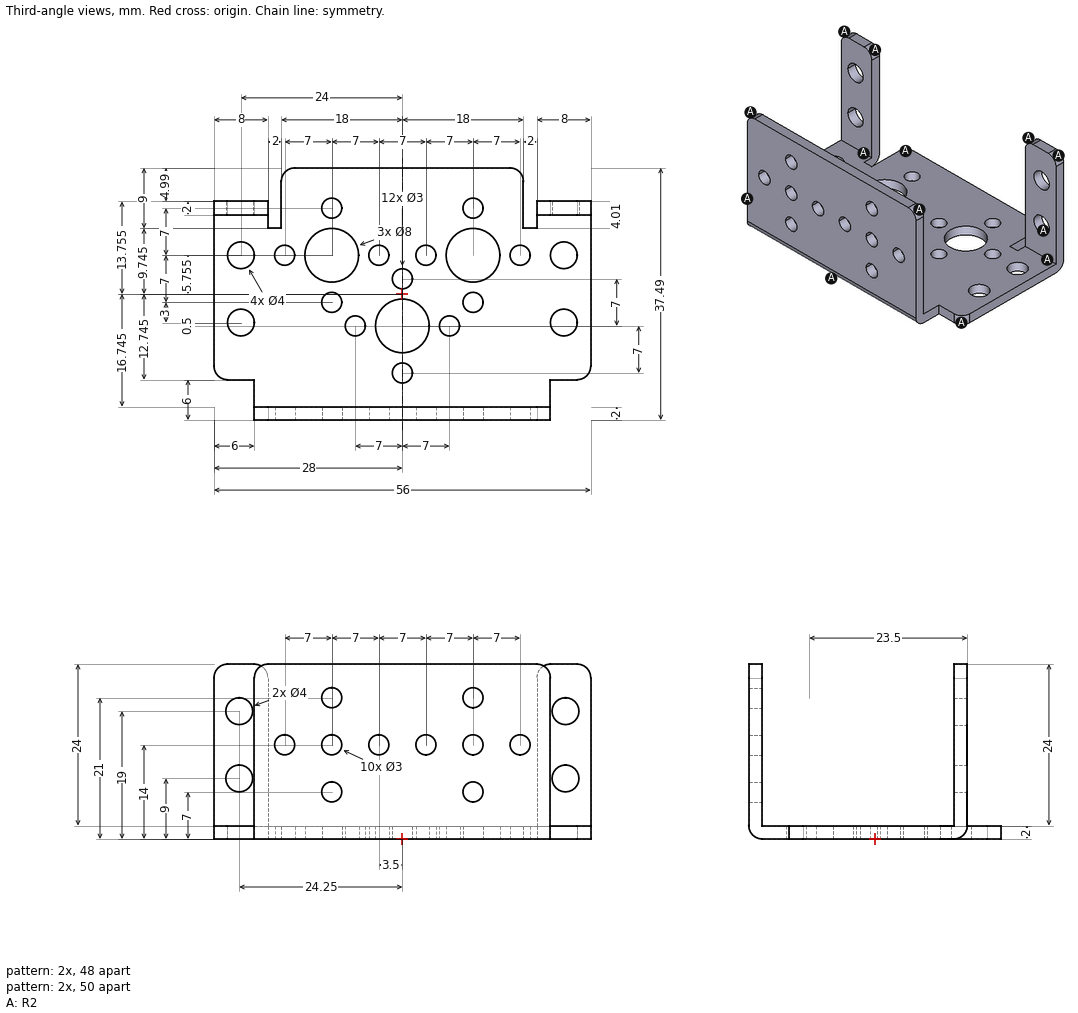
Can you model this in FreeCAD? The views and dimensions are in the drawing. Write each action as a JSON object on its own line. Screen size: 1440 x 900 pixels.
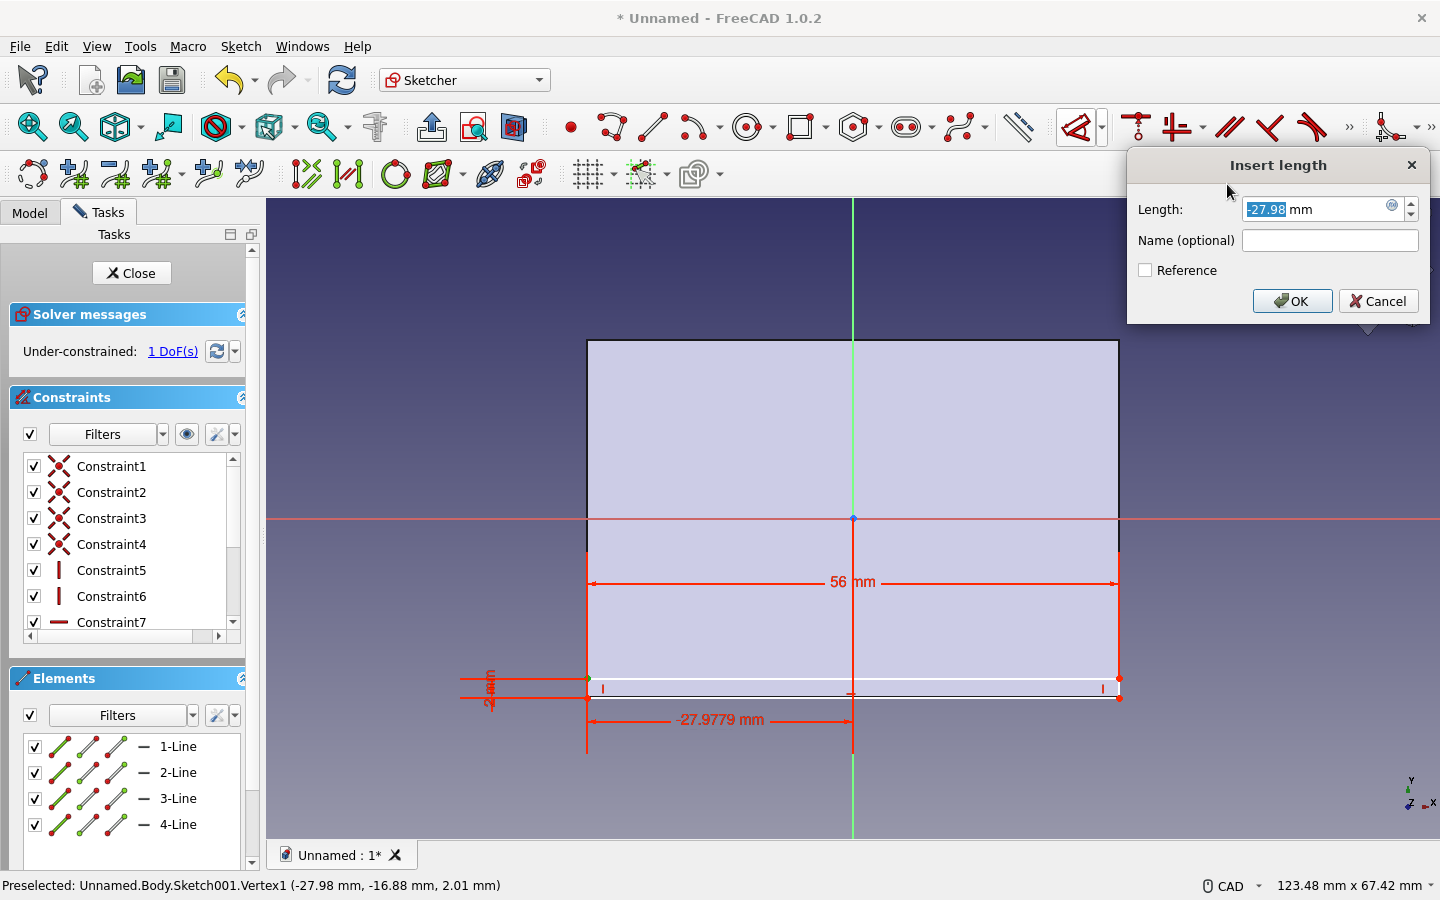
{"action": "type", "text": "-28"}
{"action": "key", "text": "Return"}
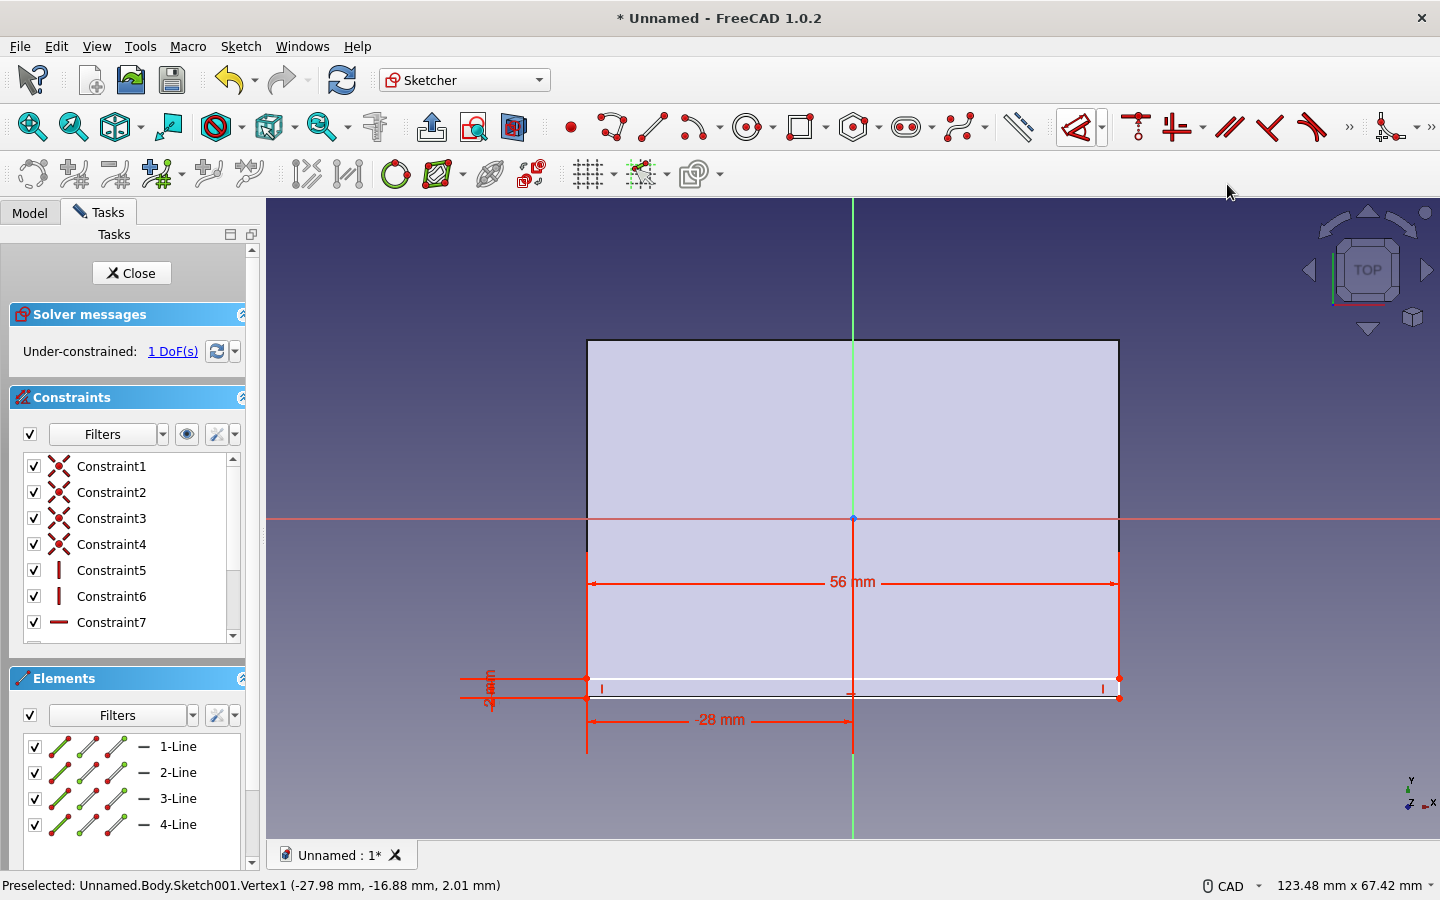
{"action": "left_click", "coordinate": [587, 679]}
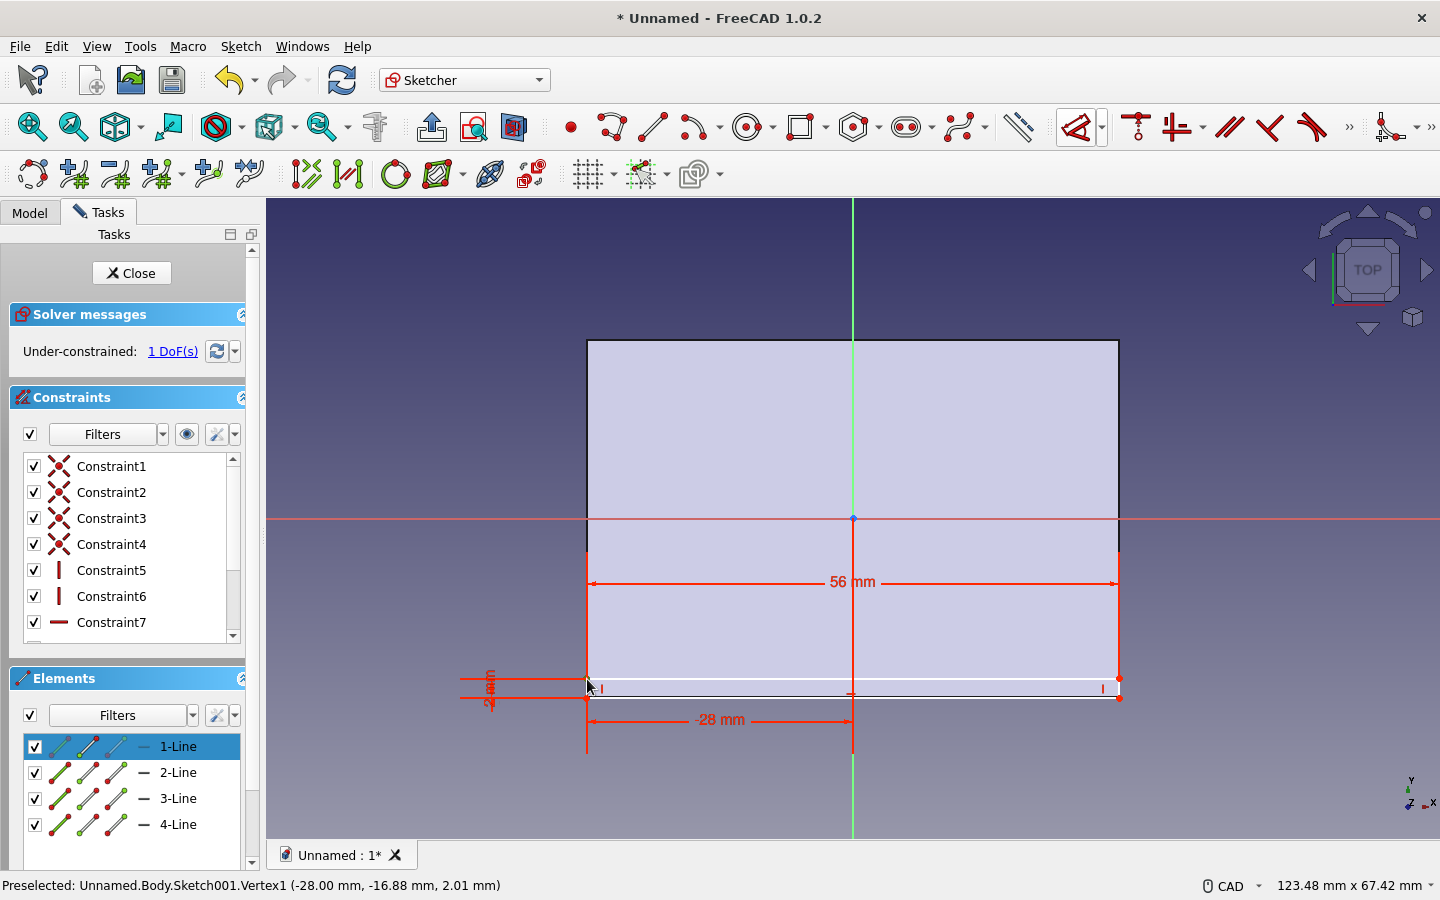
{"action": "key", "text": "i"}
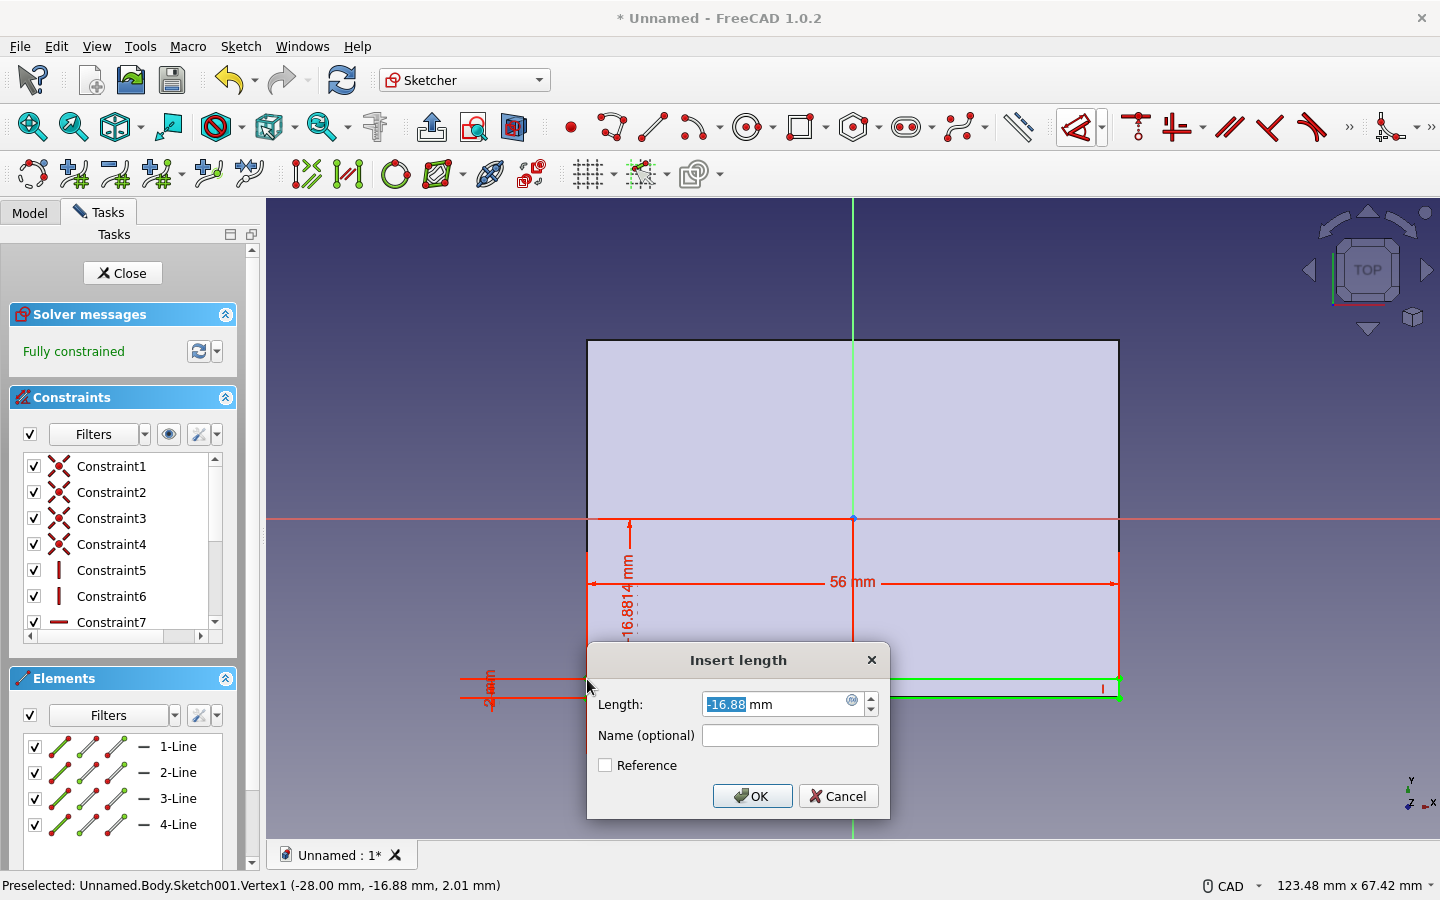
{"action": "type", "text": "-16.745"}
{"action": "key", "text": "Return"}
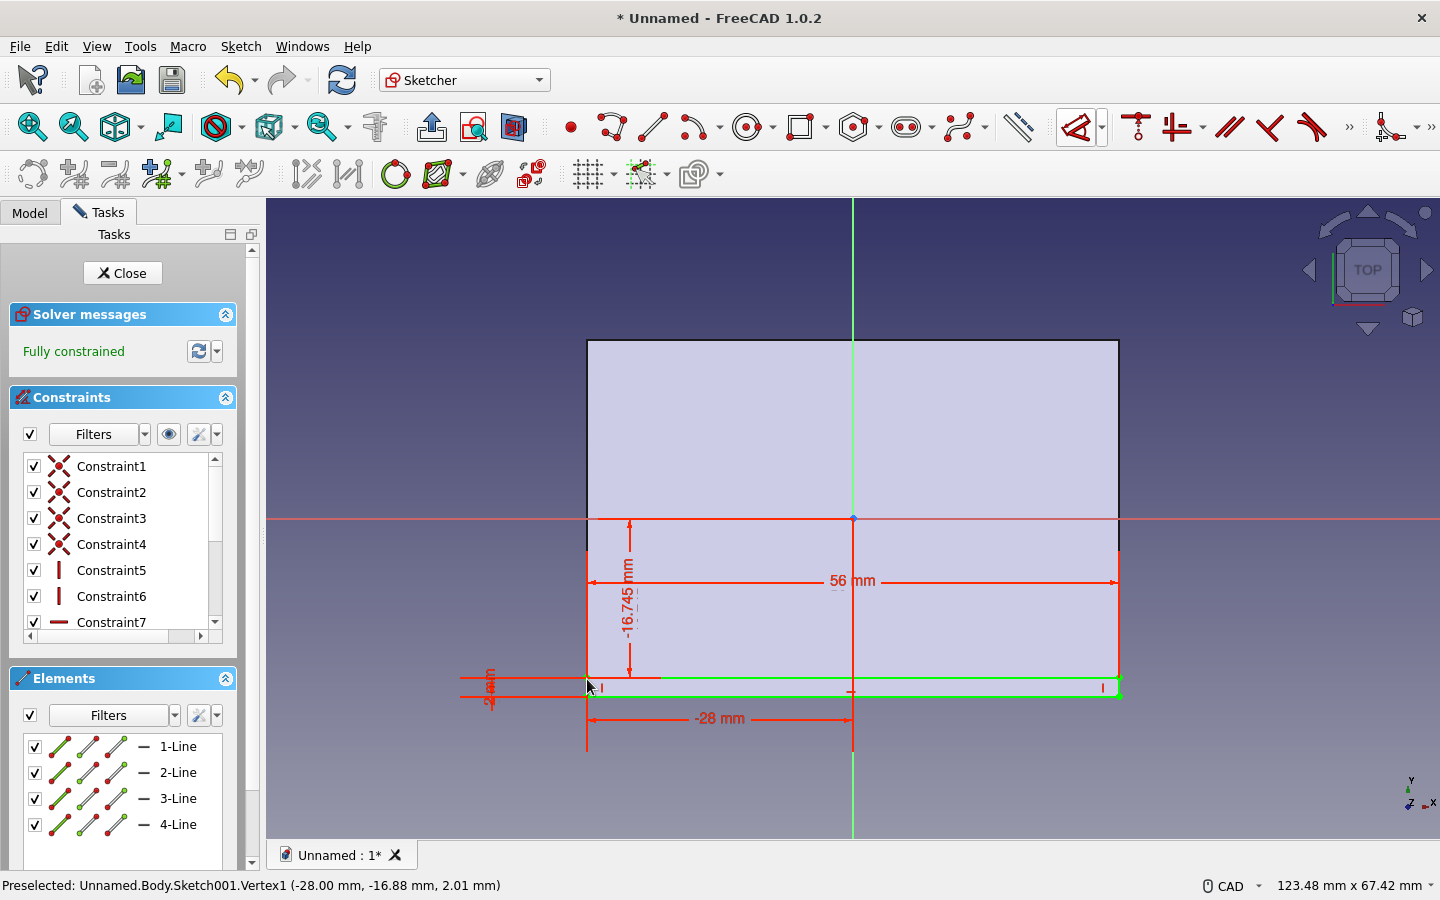
{"action": "left_click", "coordinate": [123, 273]}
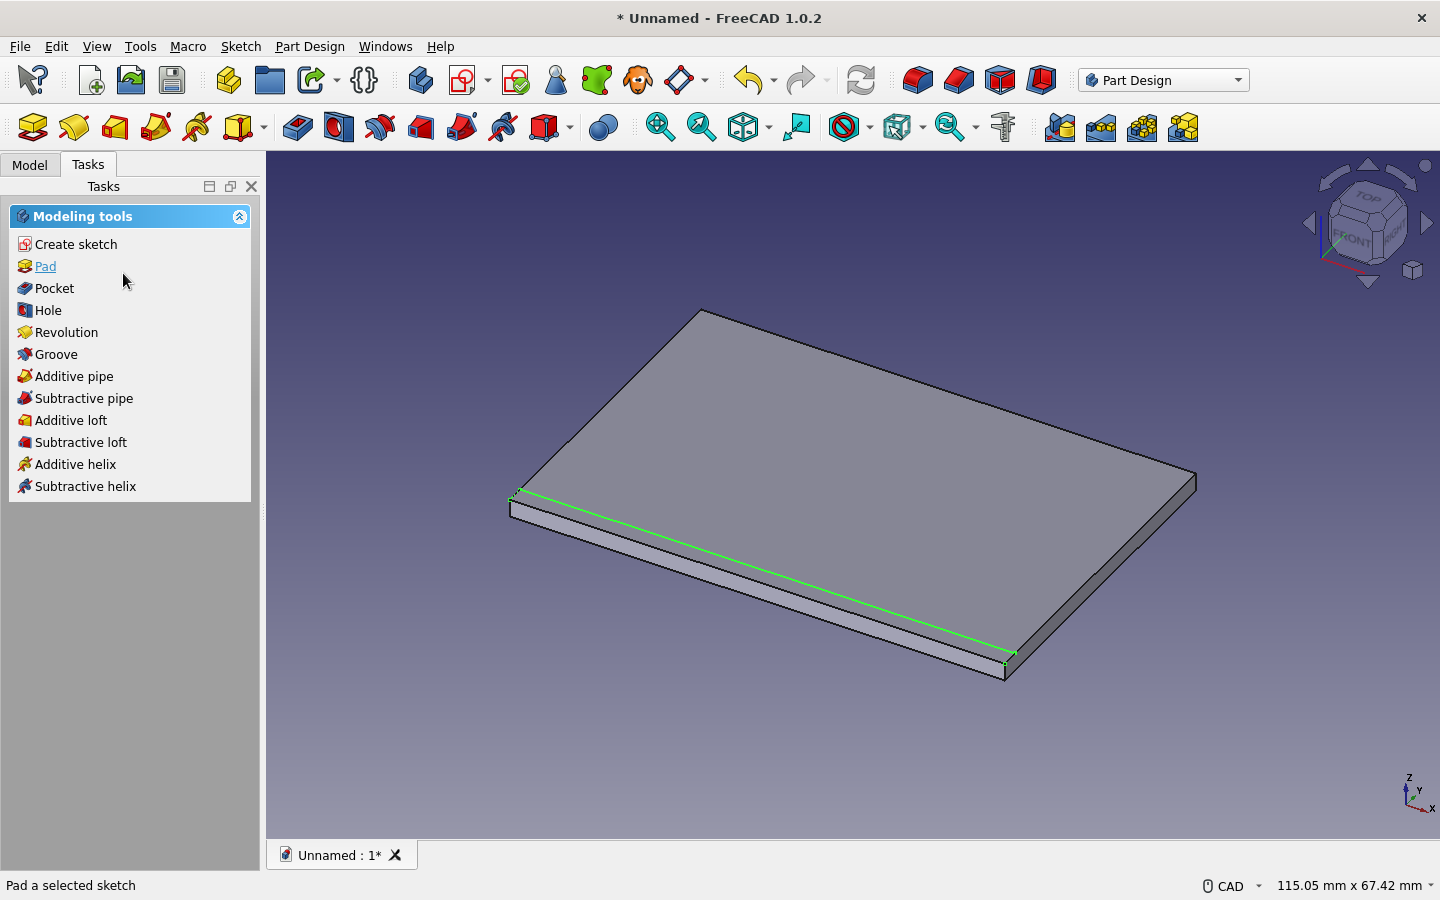
{"action": "left_click", "coordinate": [33, 128]}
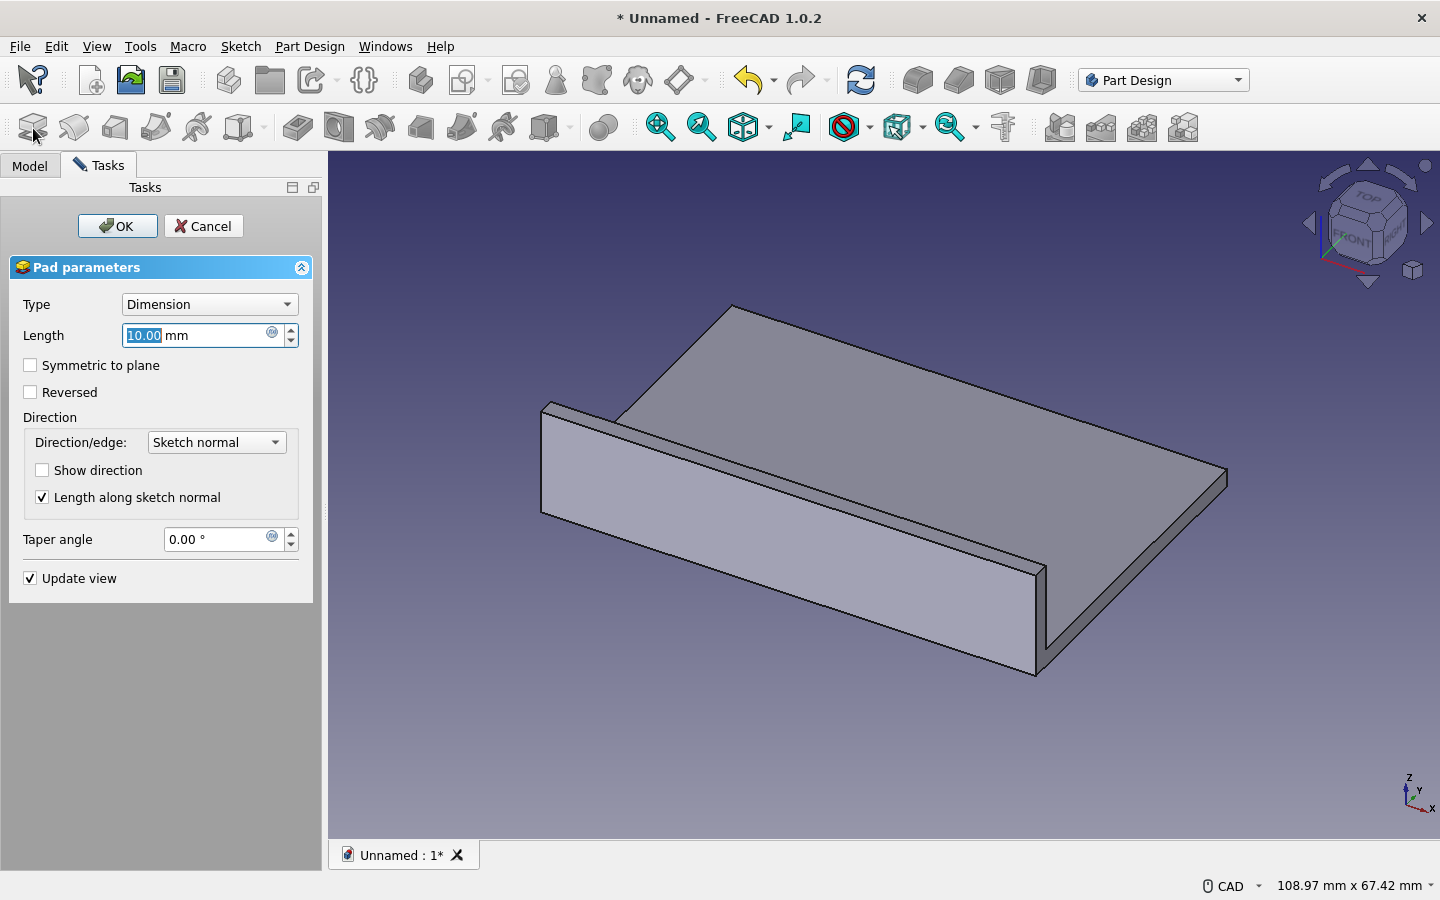
{"action": "type", "text": "24"}
{"action": "key", "text": "Tab"}